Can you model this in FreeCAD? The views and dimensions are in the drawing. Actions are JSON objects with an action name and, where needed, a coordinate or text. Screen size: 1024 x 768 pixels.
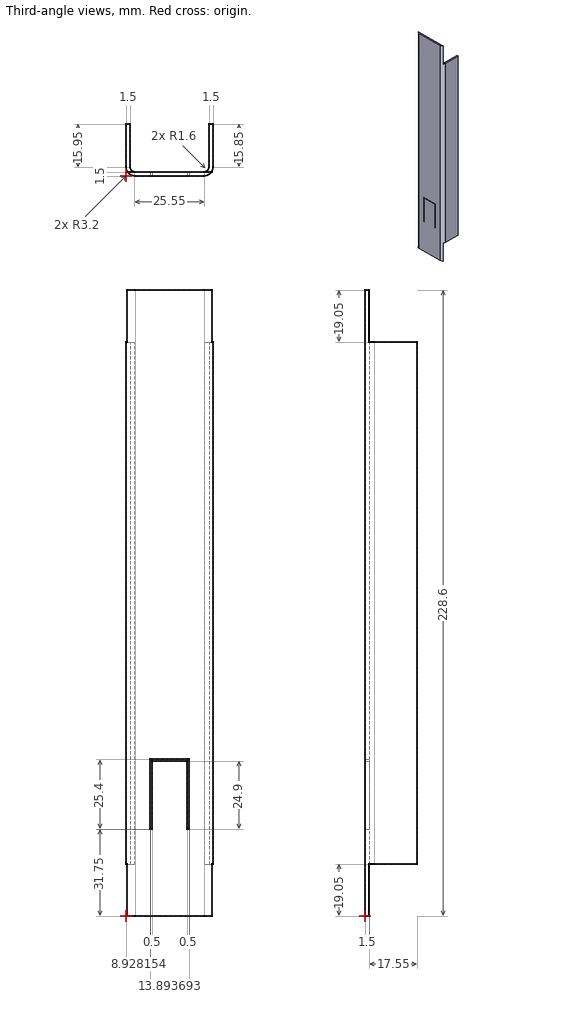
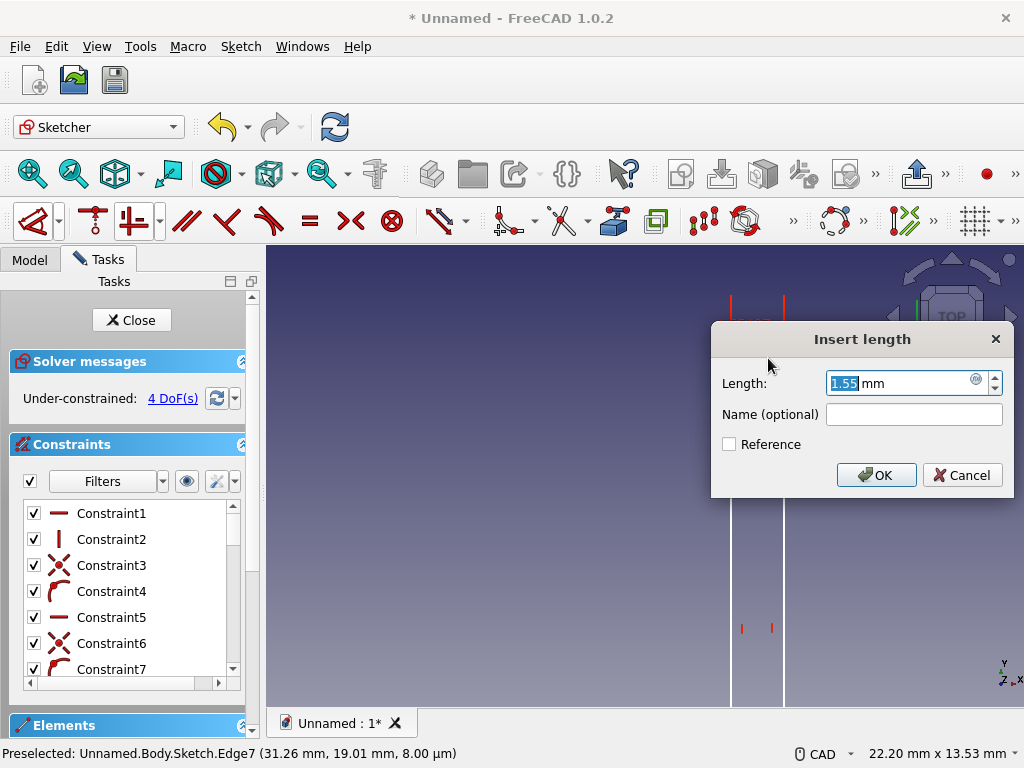
{"action": "type", "text": "1.5"}
{"action": "key", "text": "Return"}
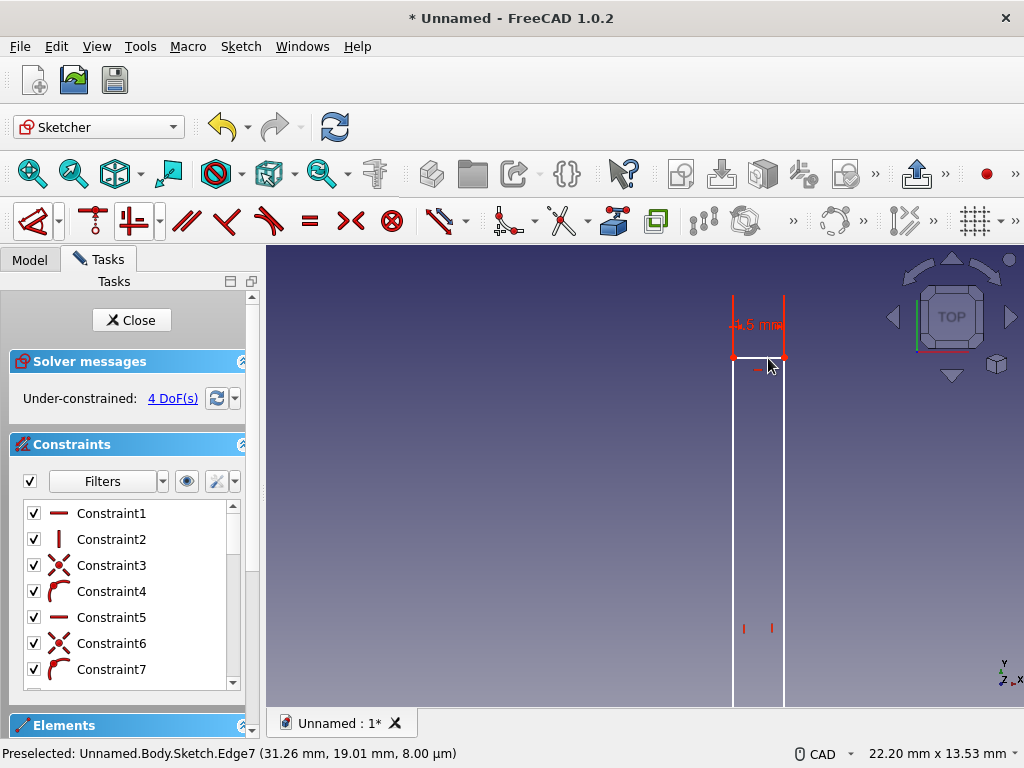
{"action": "scroll", "coordinate": [771, 357], "scroll_direction": "down", "scroll_amount": 5}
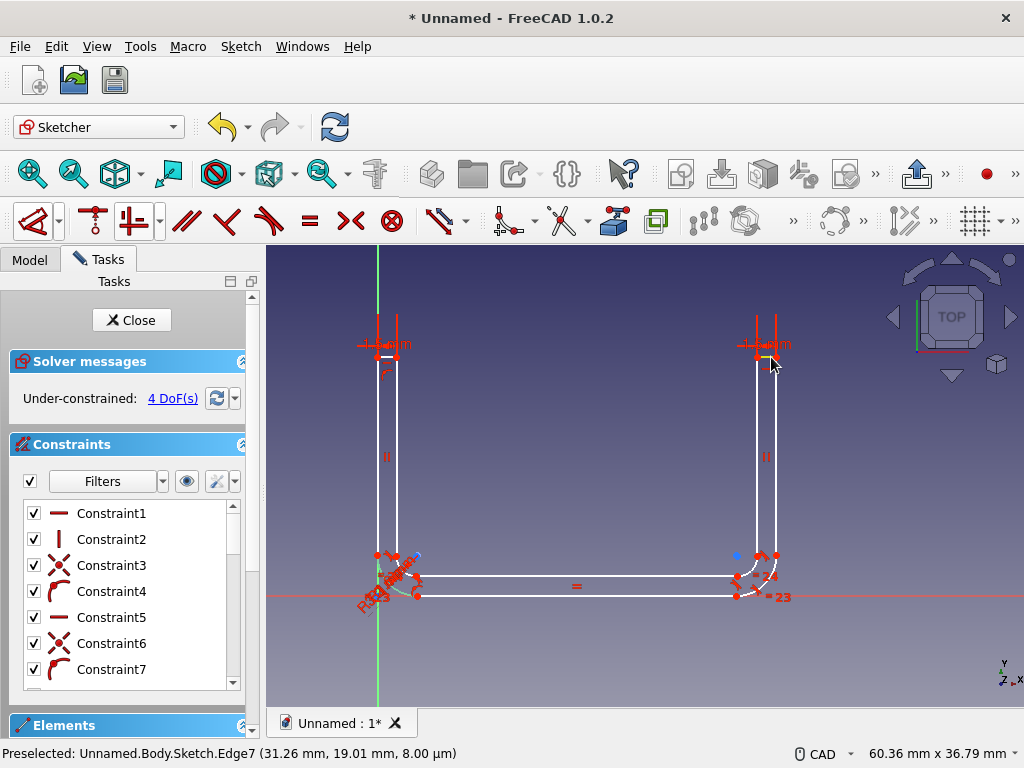
{"action": "scroll", "coordinate": [737, 576], "scroll_direction": "up", "scroll_amount": 4}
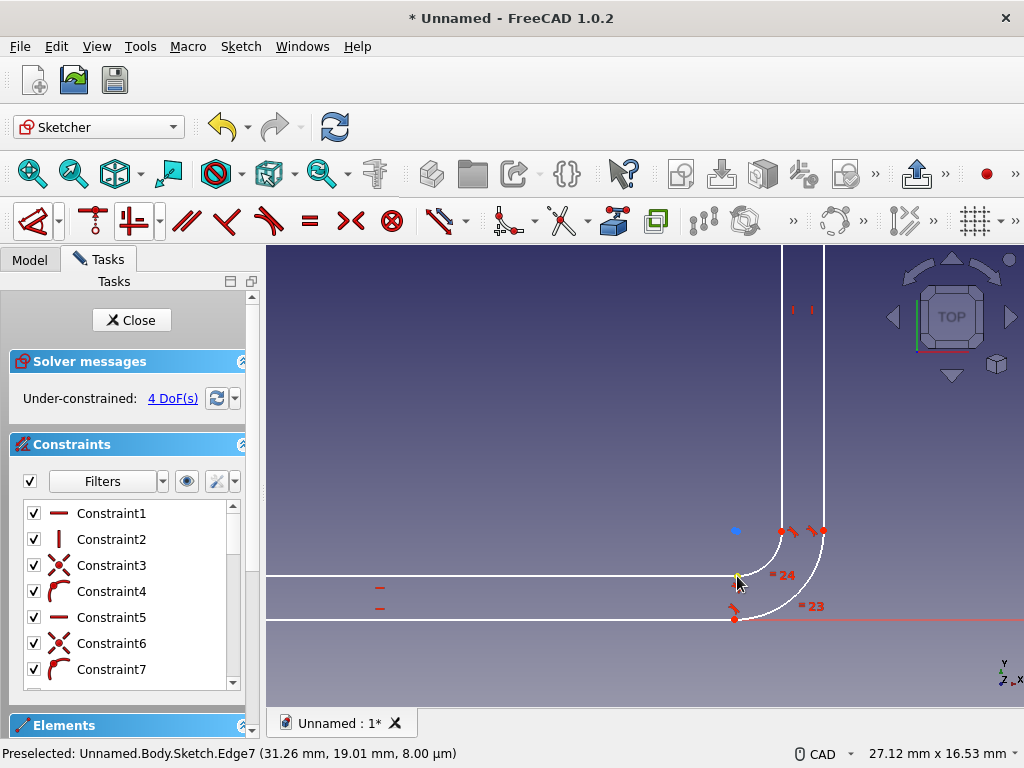
{"action": "left_click", "coordinate": [737, 576]}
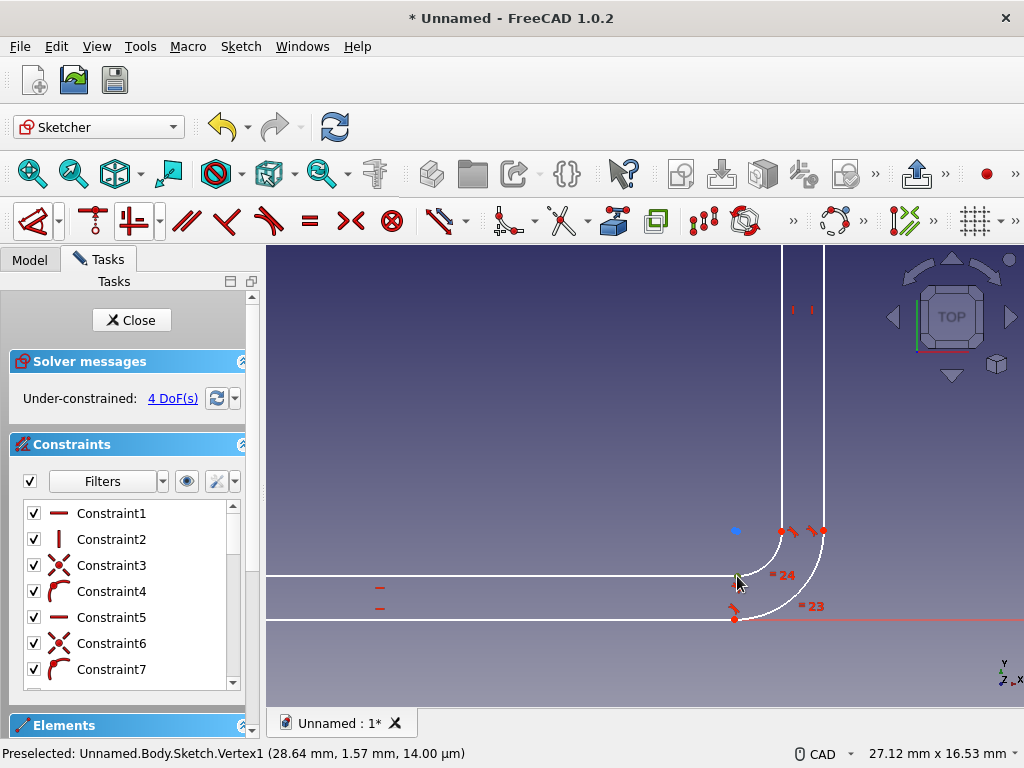
{"action": "left_click", "coordinate": [58, 222]}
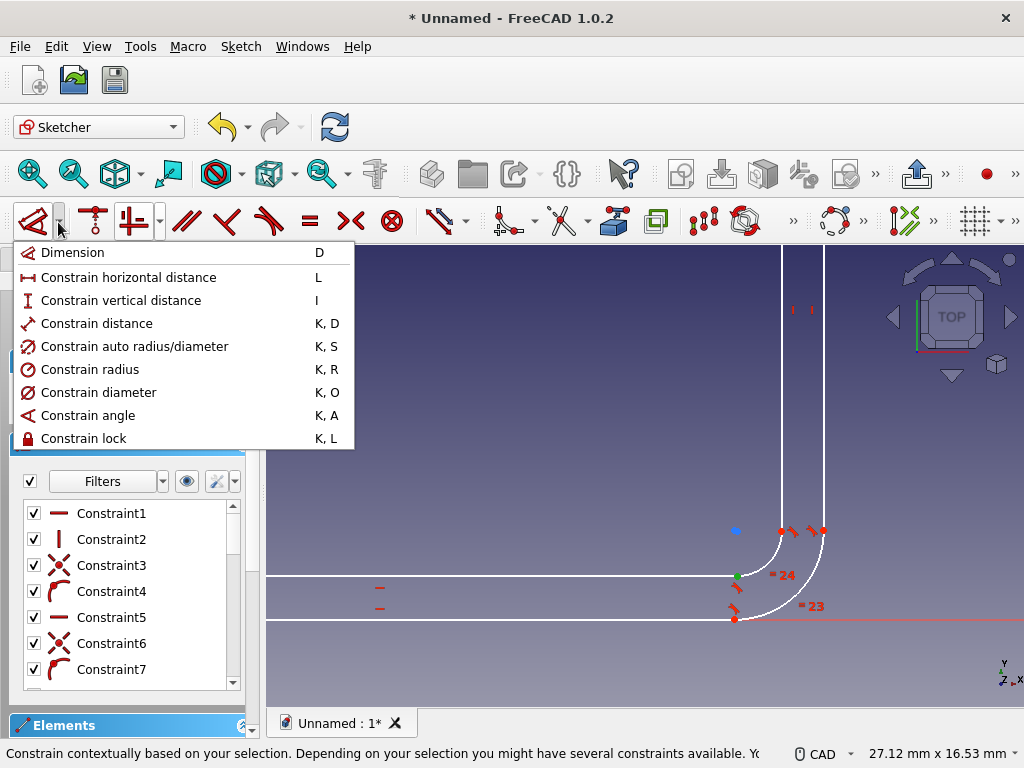
{"action": "left_click", "coordinate": [184, 300]}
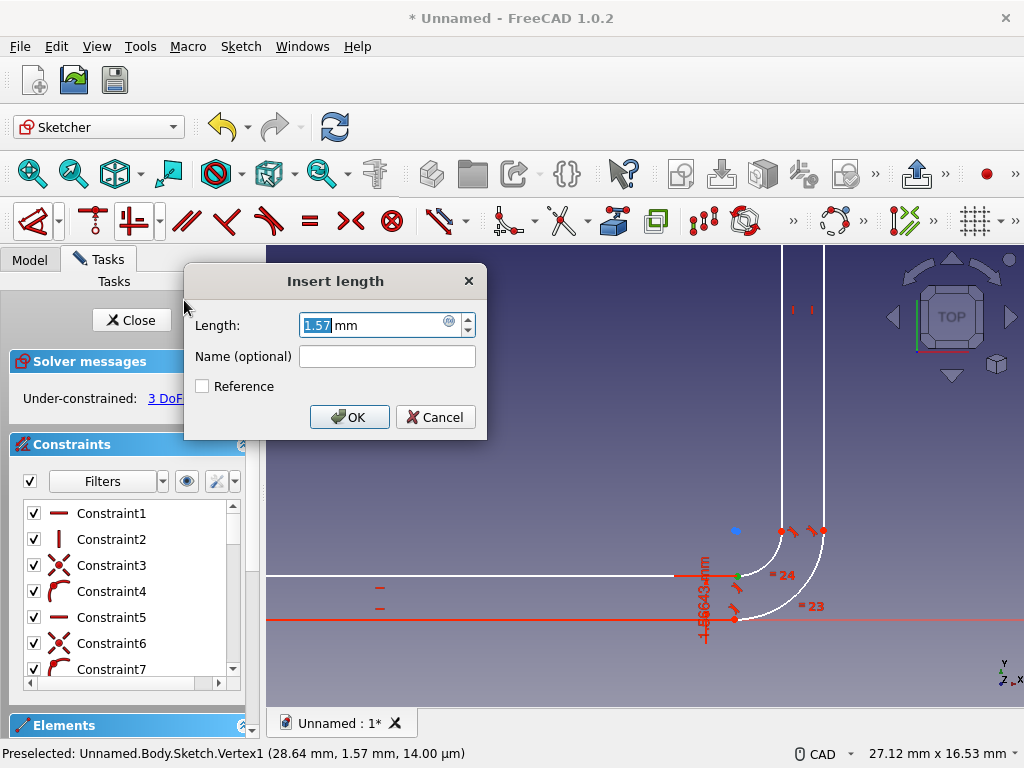
{"action": "type", "text": "1.5"}
{"action": "key", "text": "Return"}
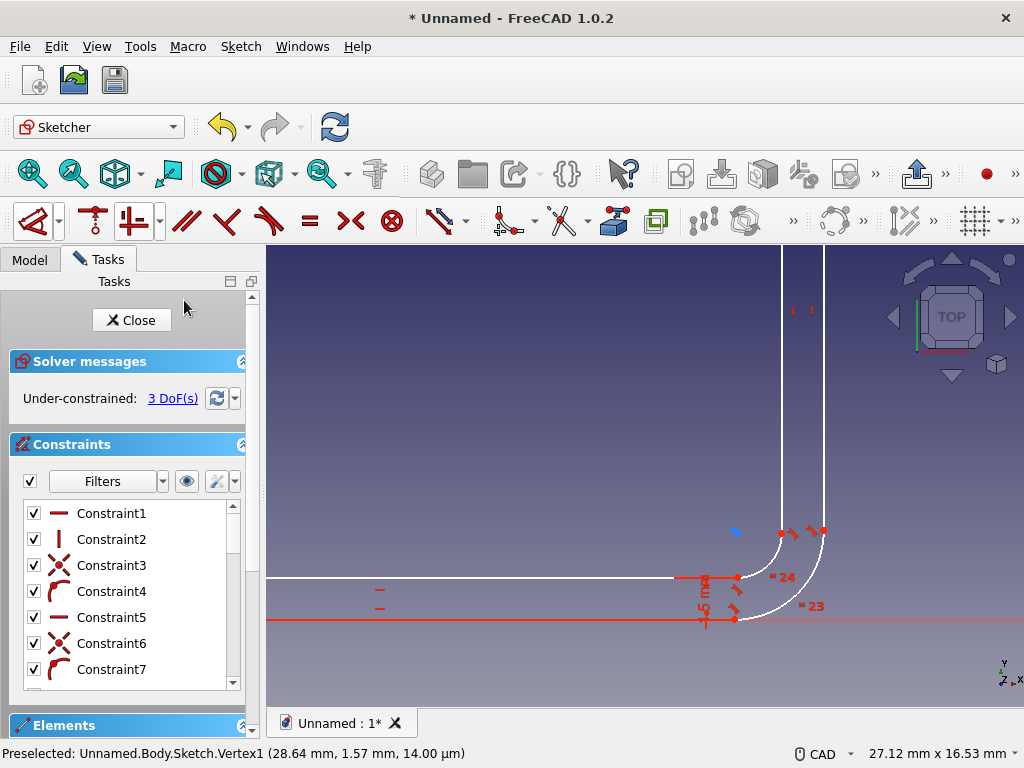
{"action": "left_click", "coordinate": [523, 578]}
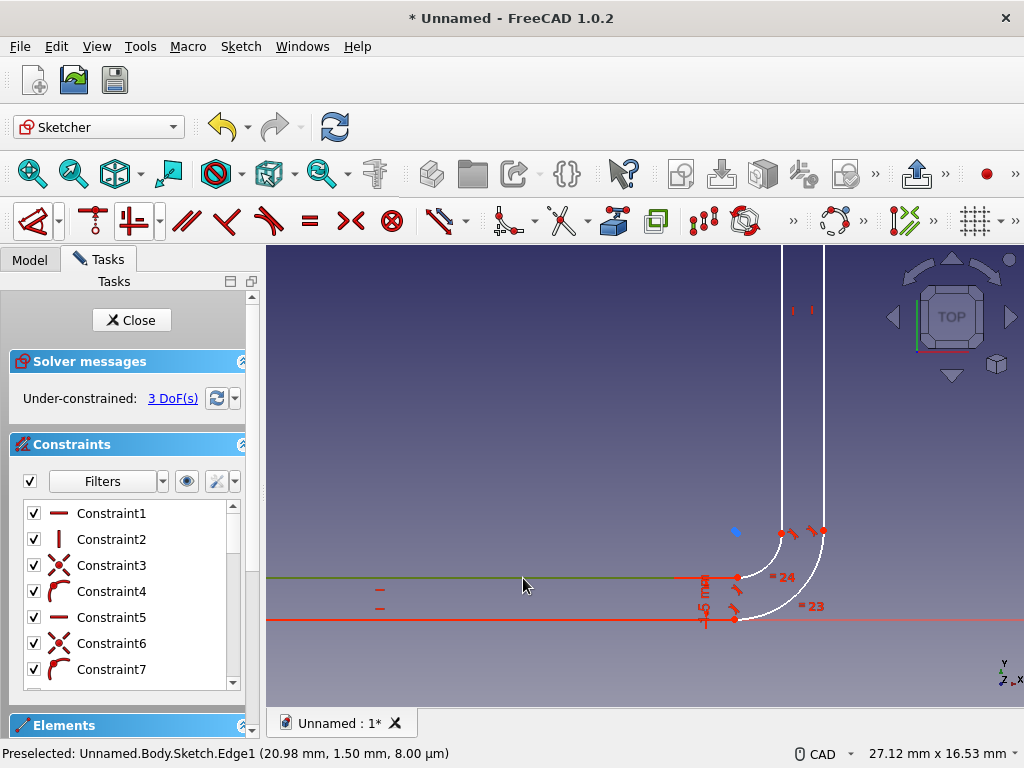
{"action": "left_click", "coordinate": [58, 222]}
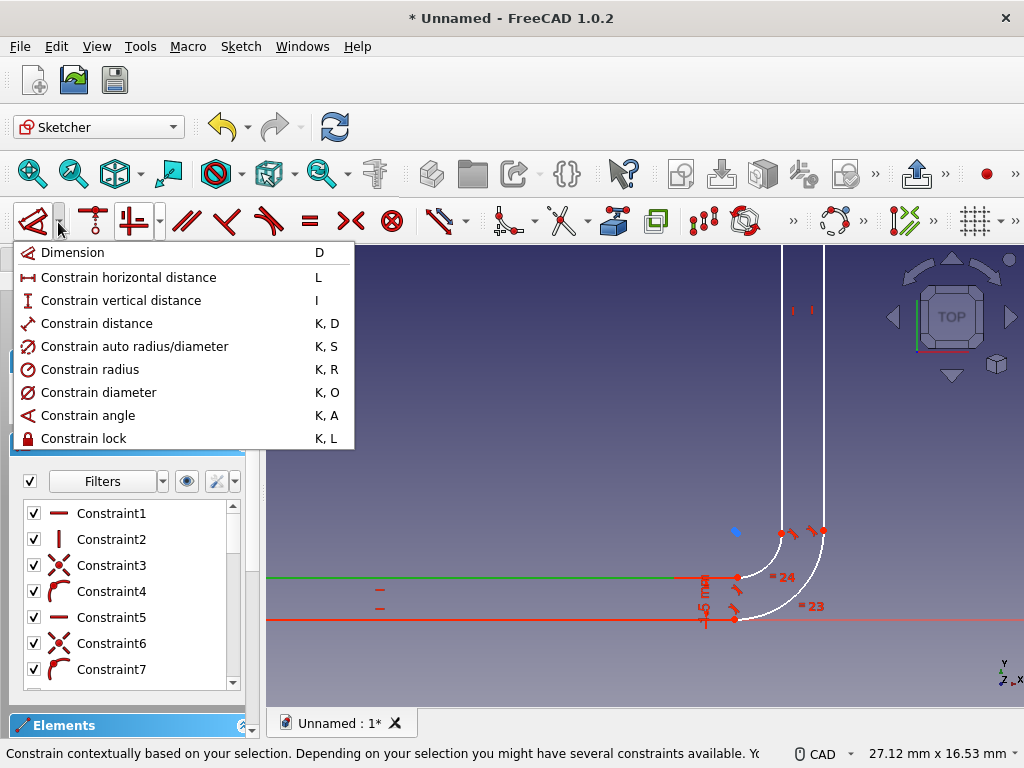
{"action": "left_click", "coordinate": [184, 278]}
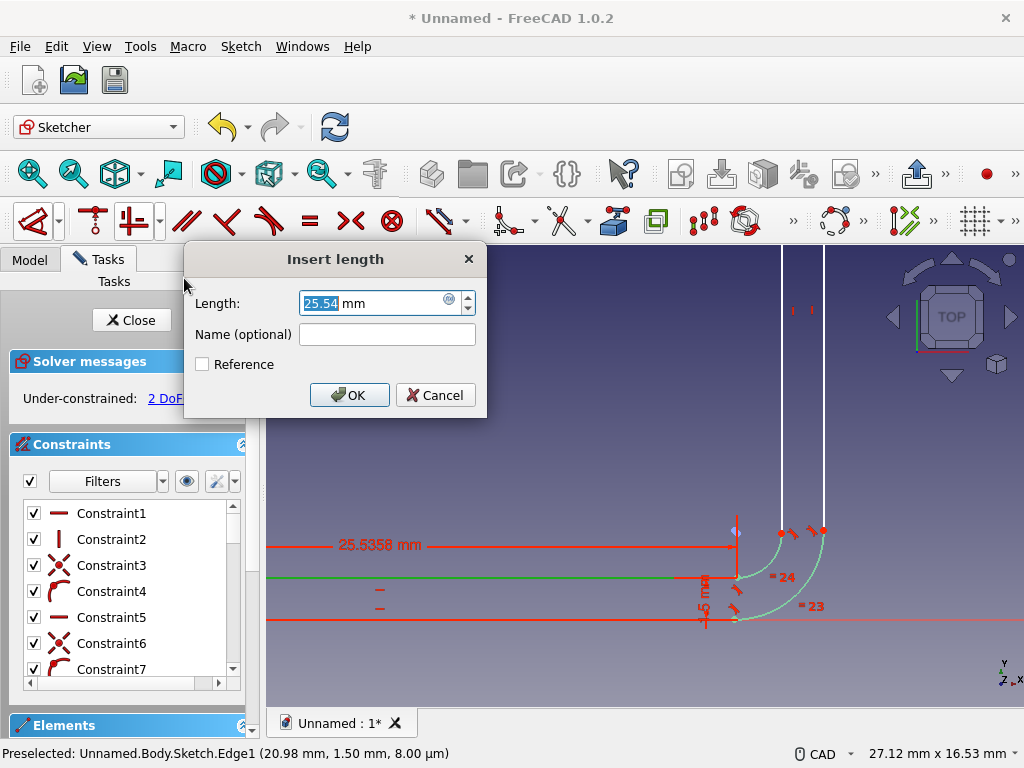
{"action": "type", "text": "25.55"}
{"action": "key", "text": "Return"}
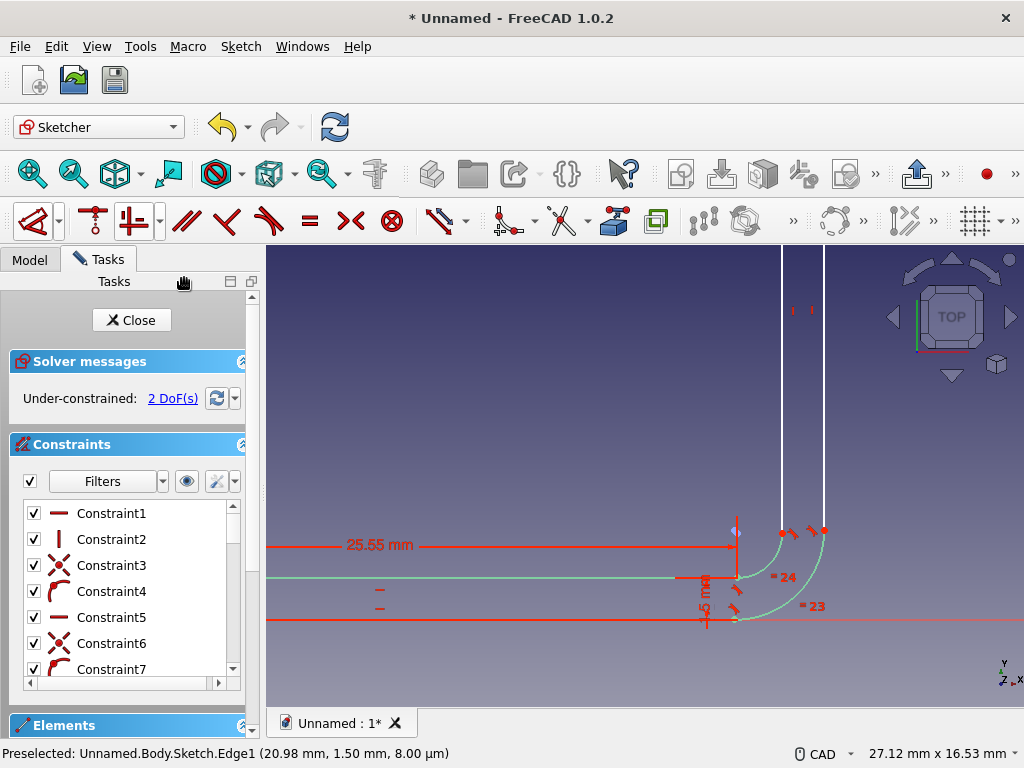
{"action": "scroll", "coordinate": [736, 576], "scroll_direction": "down", "scroll_amount": 4}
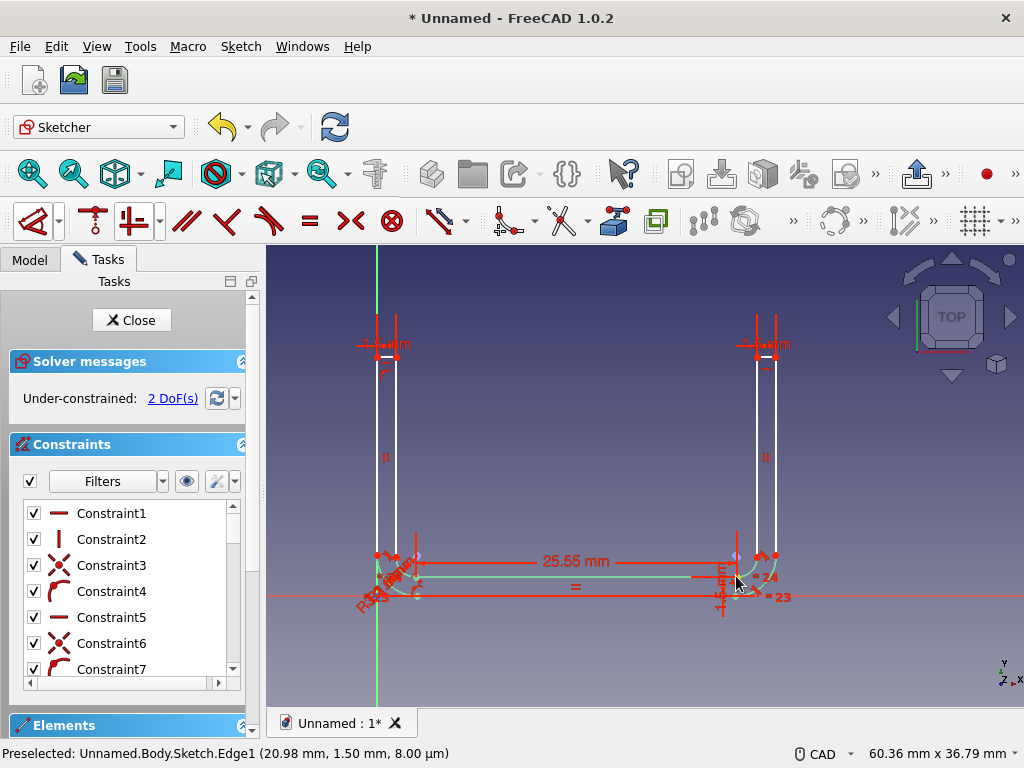
{"action": "left_click", "coordinate": [396, 497]}